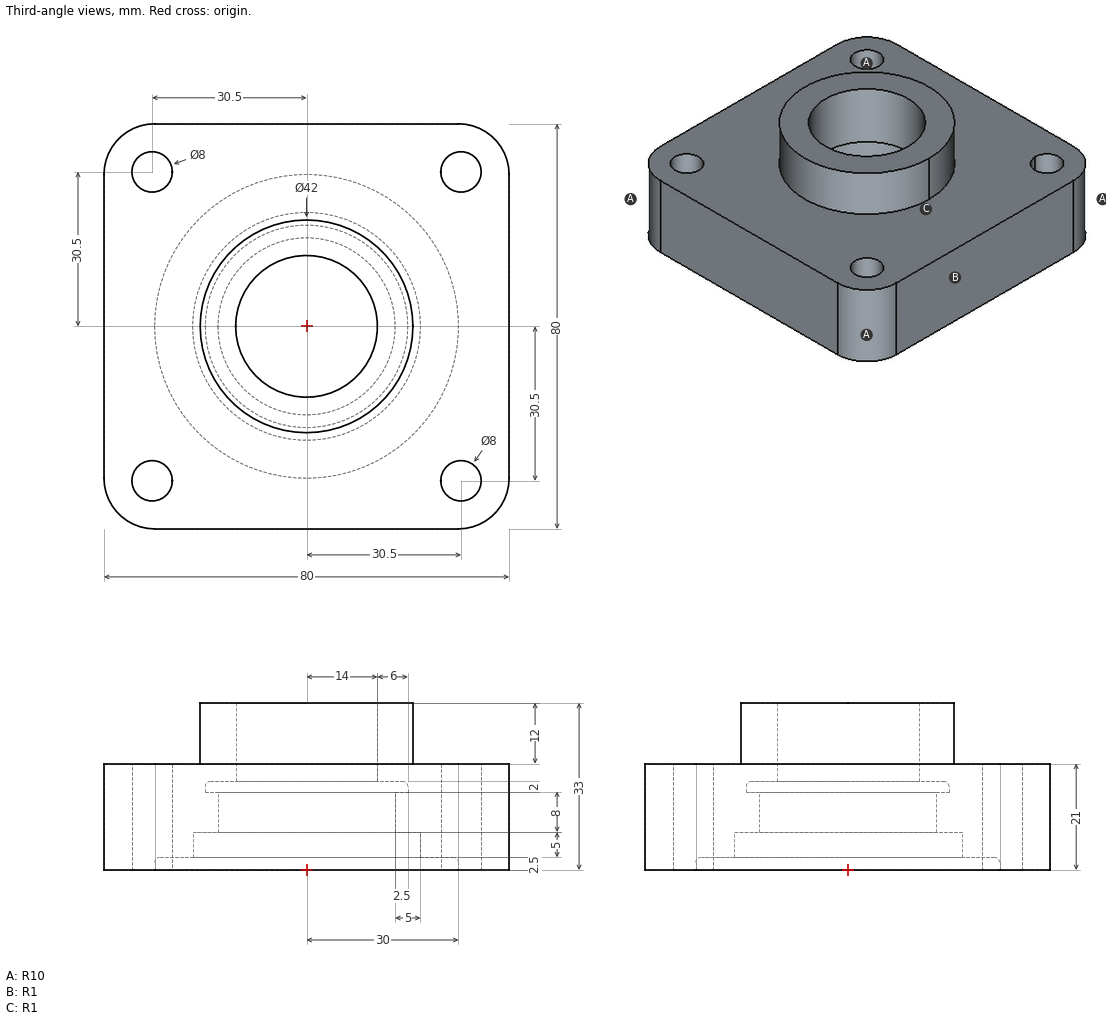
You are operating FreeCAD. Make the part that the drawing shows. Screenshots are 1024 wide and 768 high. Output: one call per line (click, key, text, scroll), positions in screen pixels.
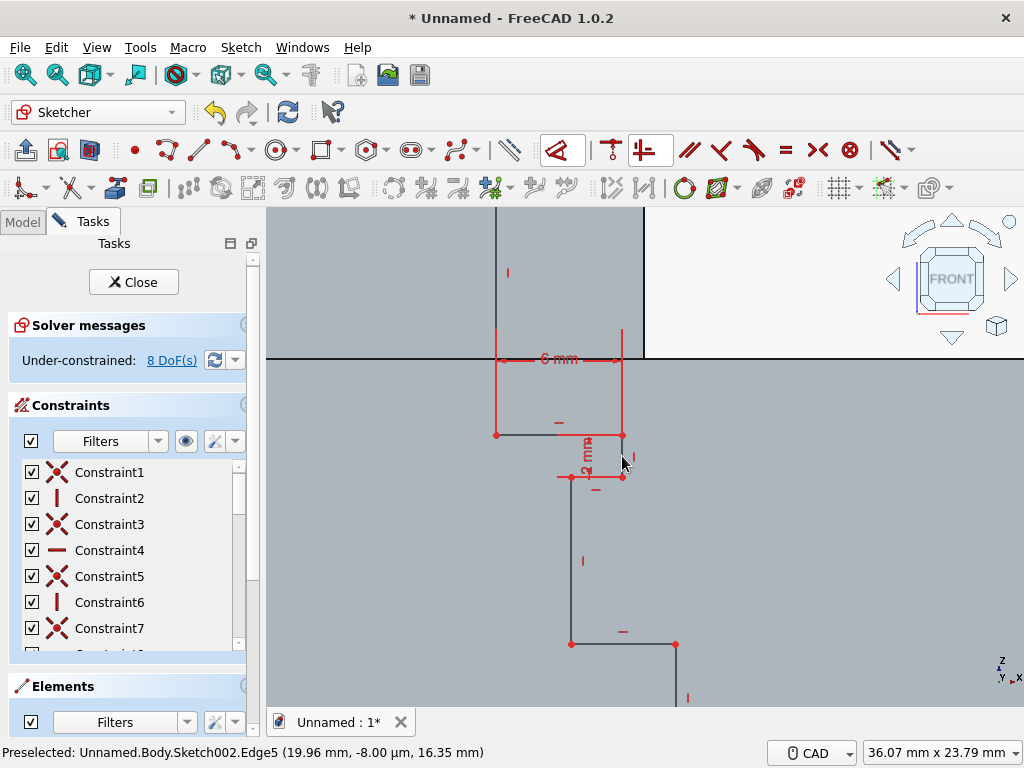
click(571, 527)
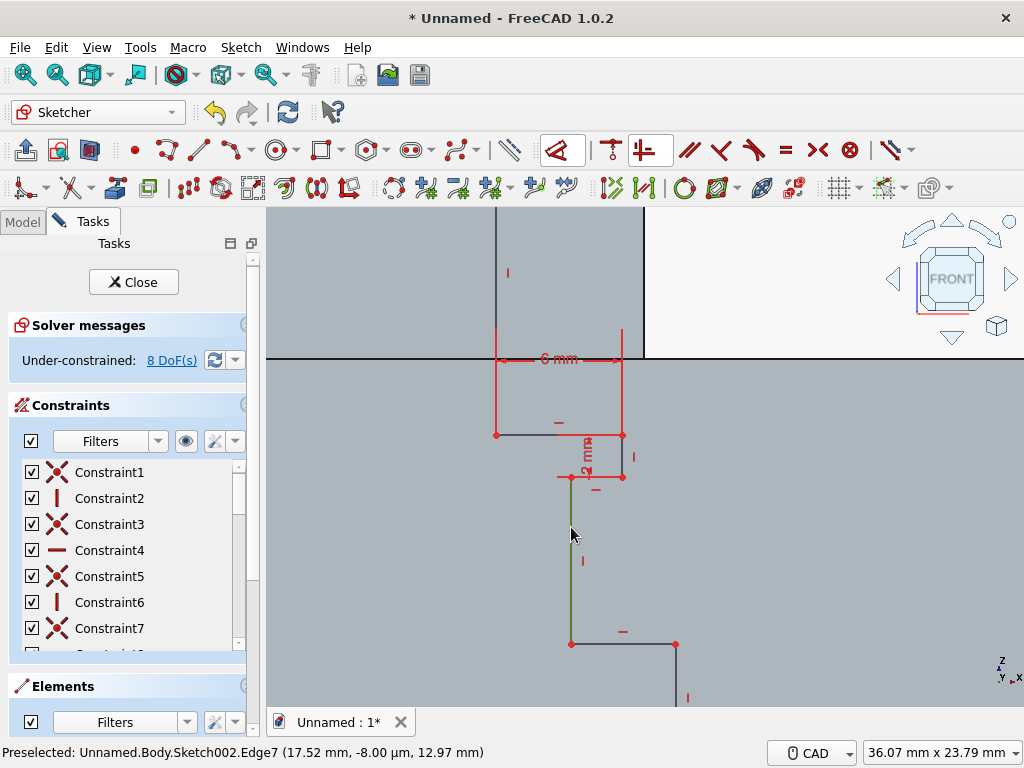
click(580, 150)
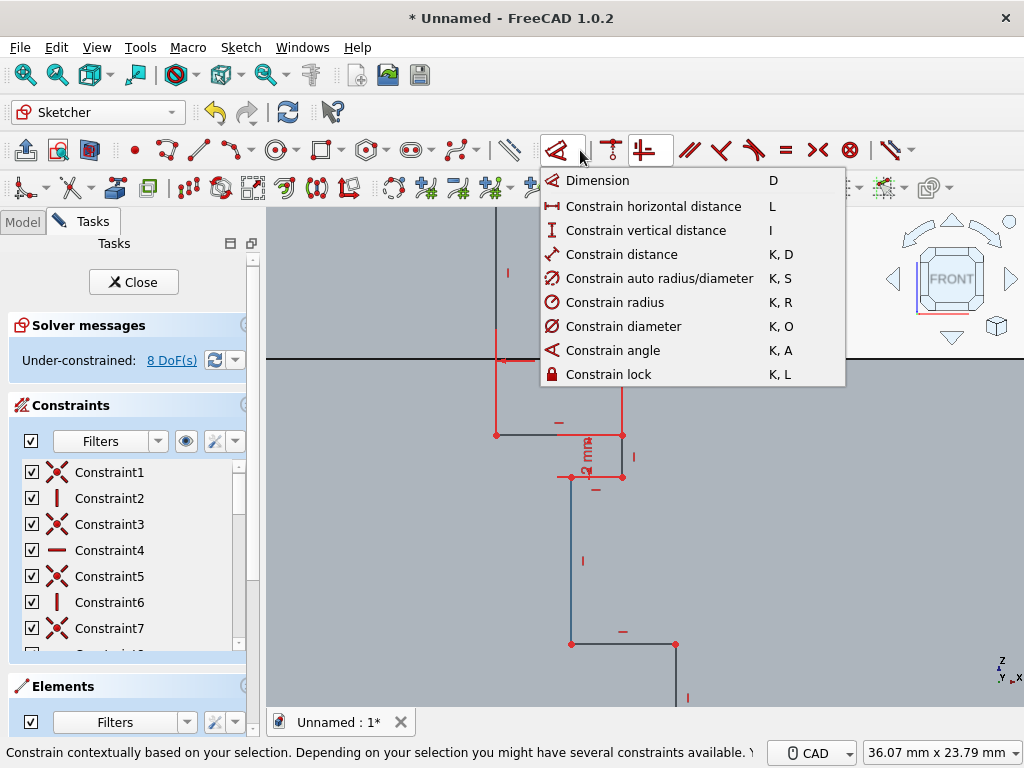
click(693, 230)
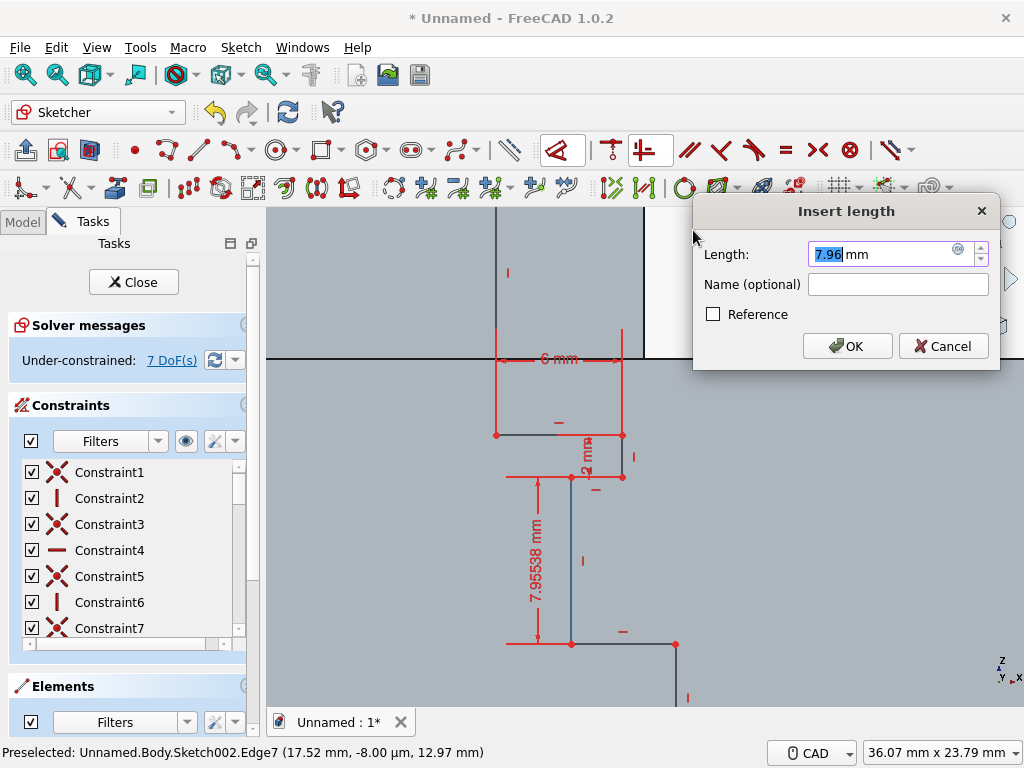
text(8)
key(Return)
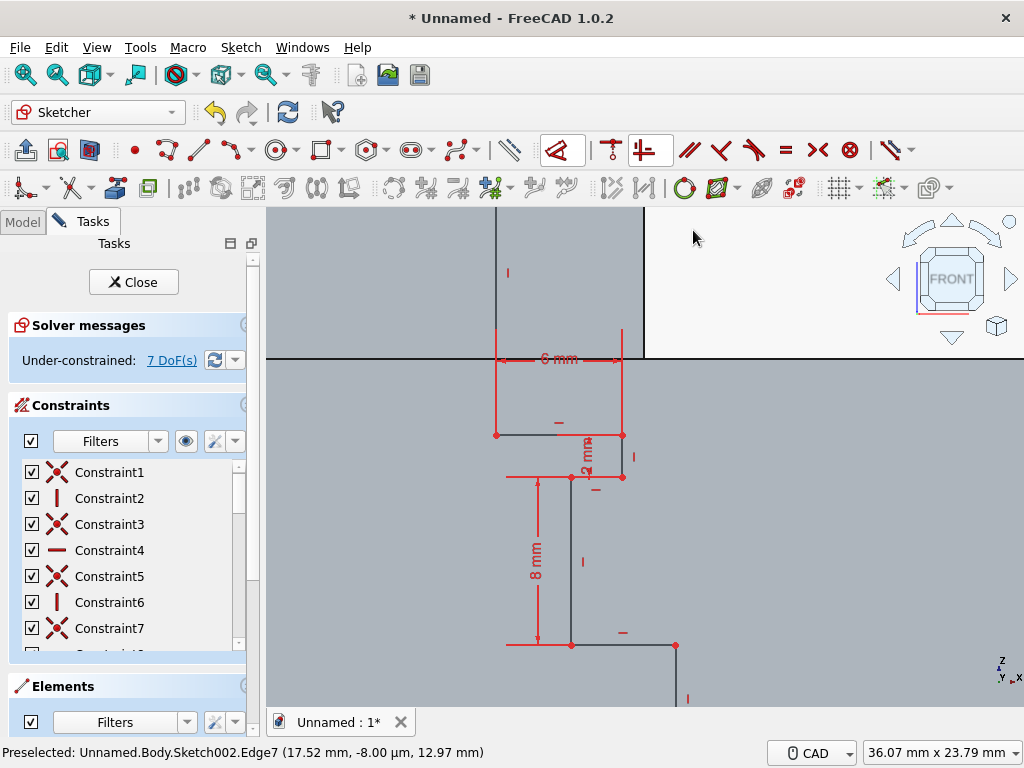
click(603, 645)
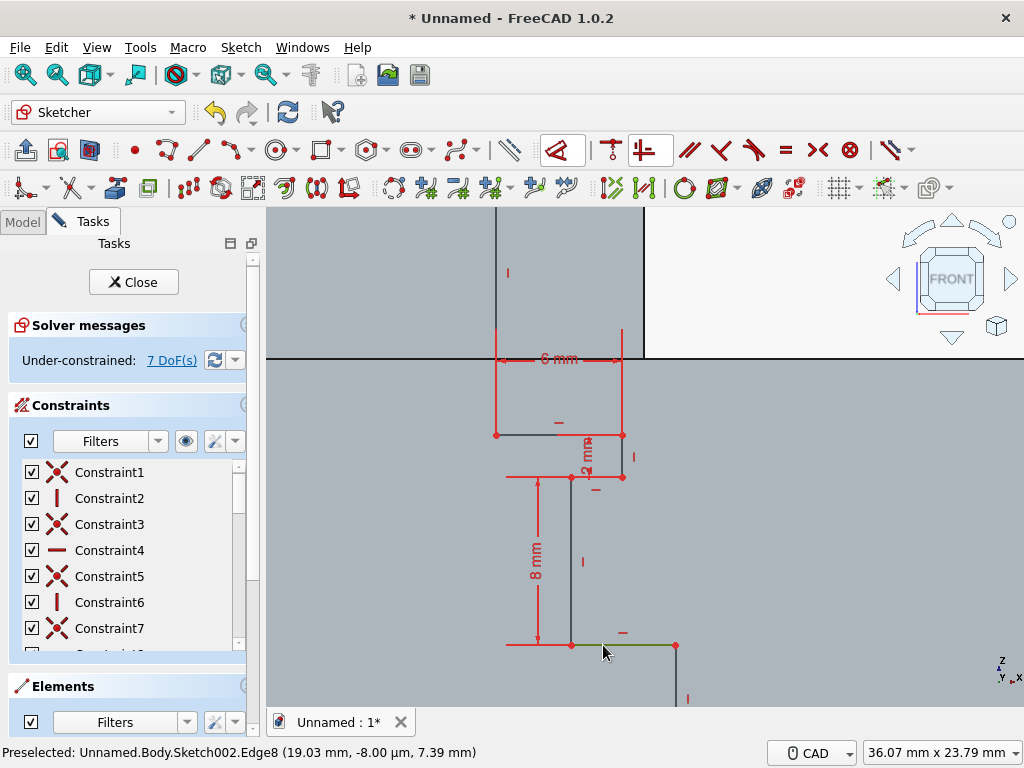
key(l)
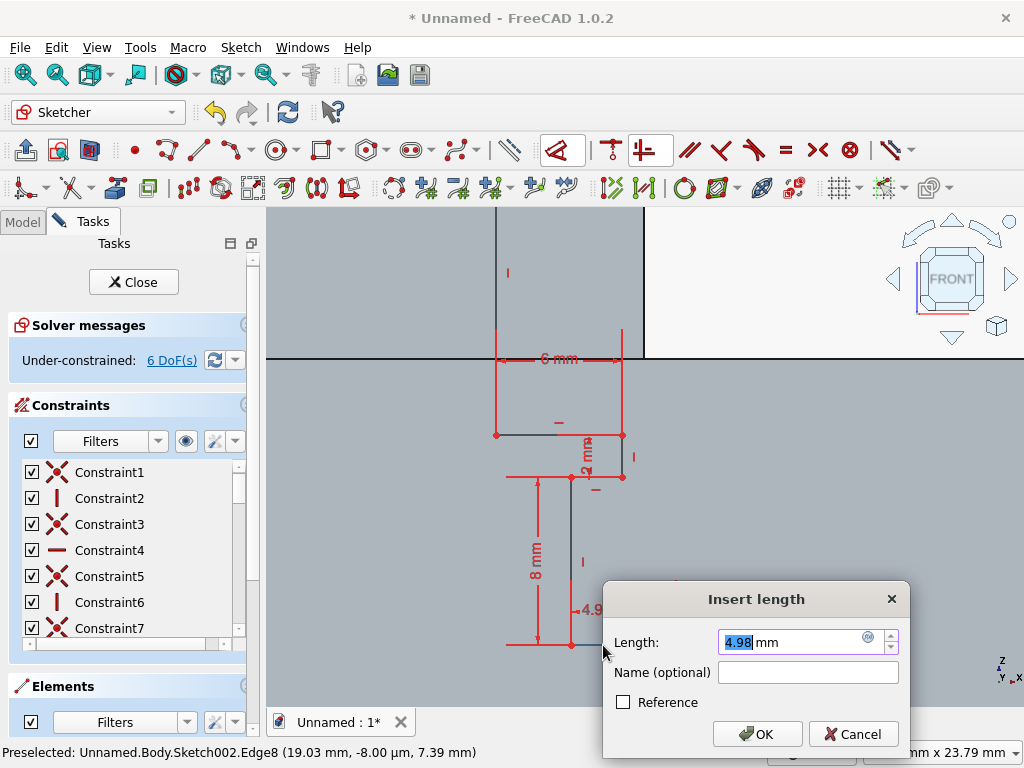
text(5)
key(Return)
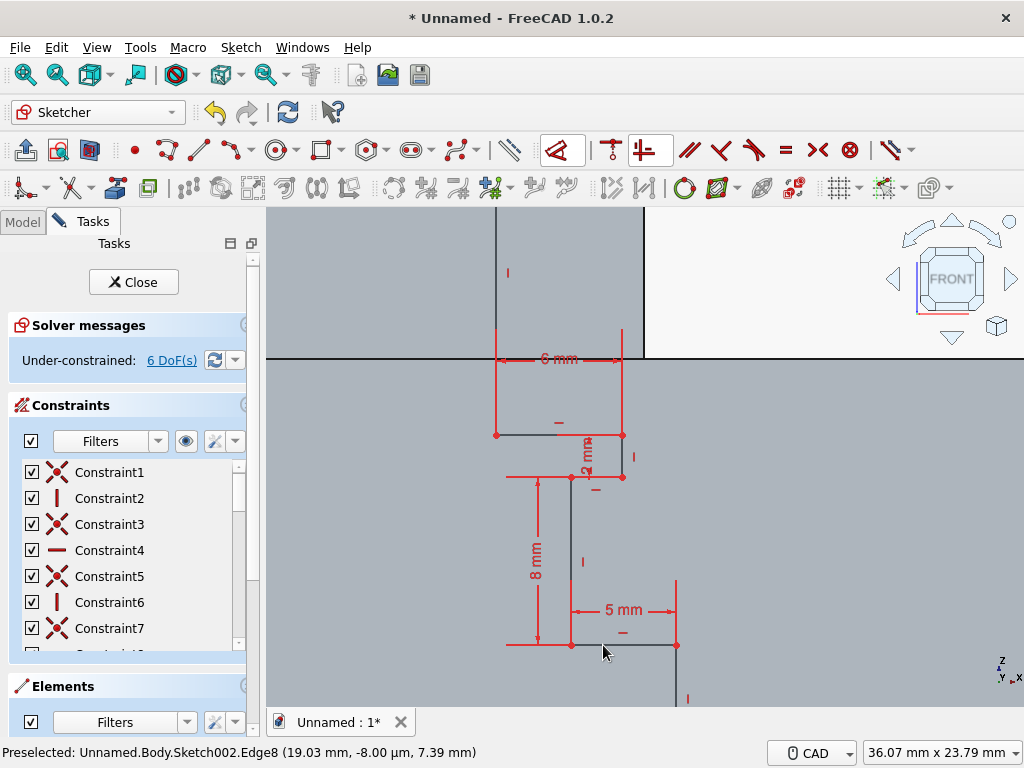
click(676, 677)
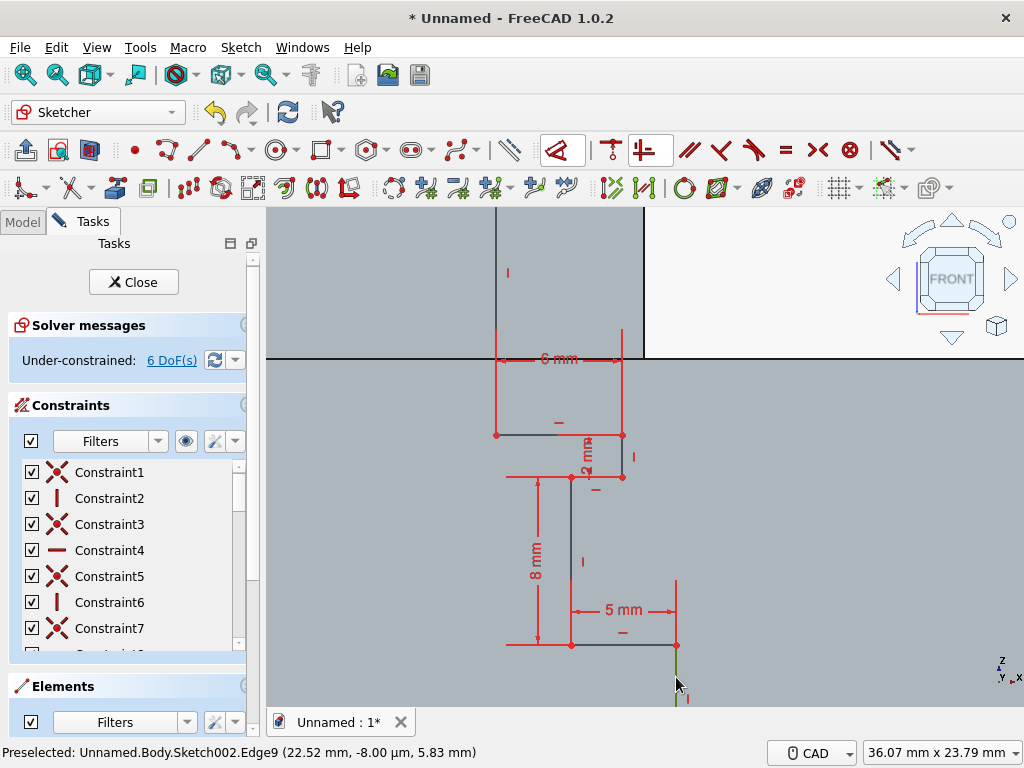
key(i)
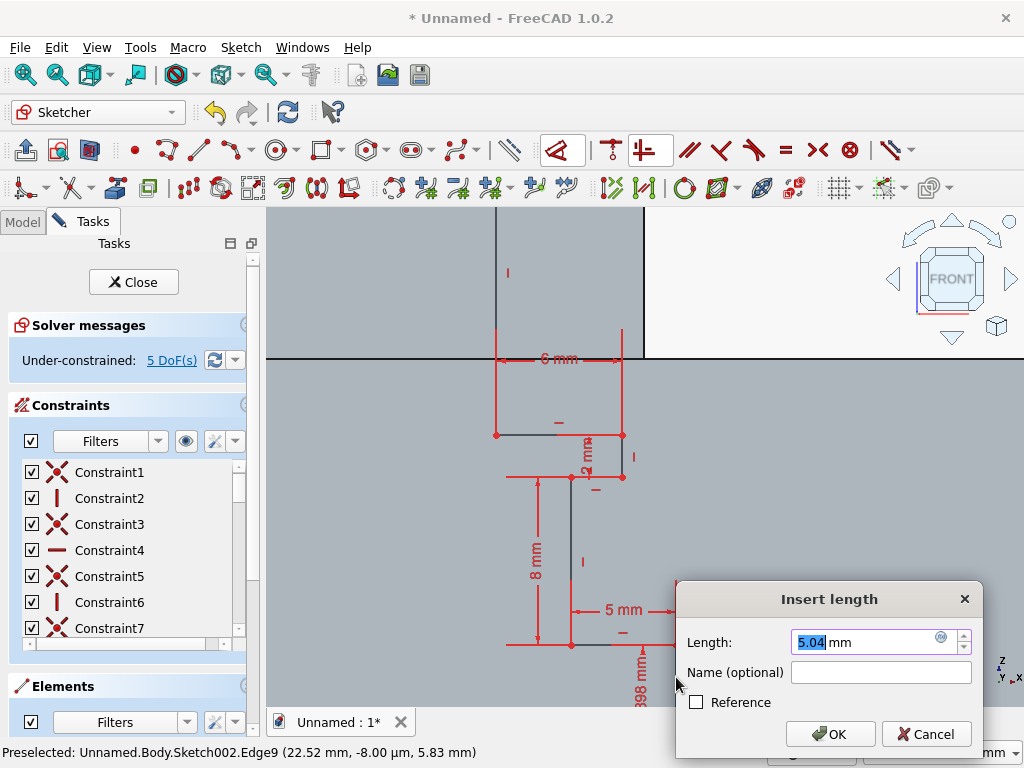
text(5)
key(Return)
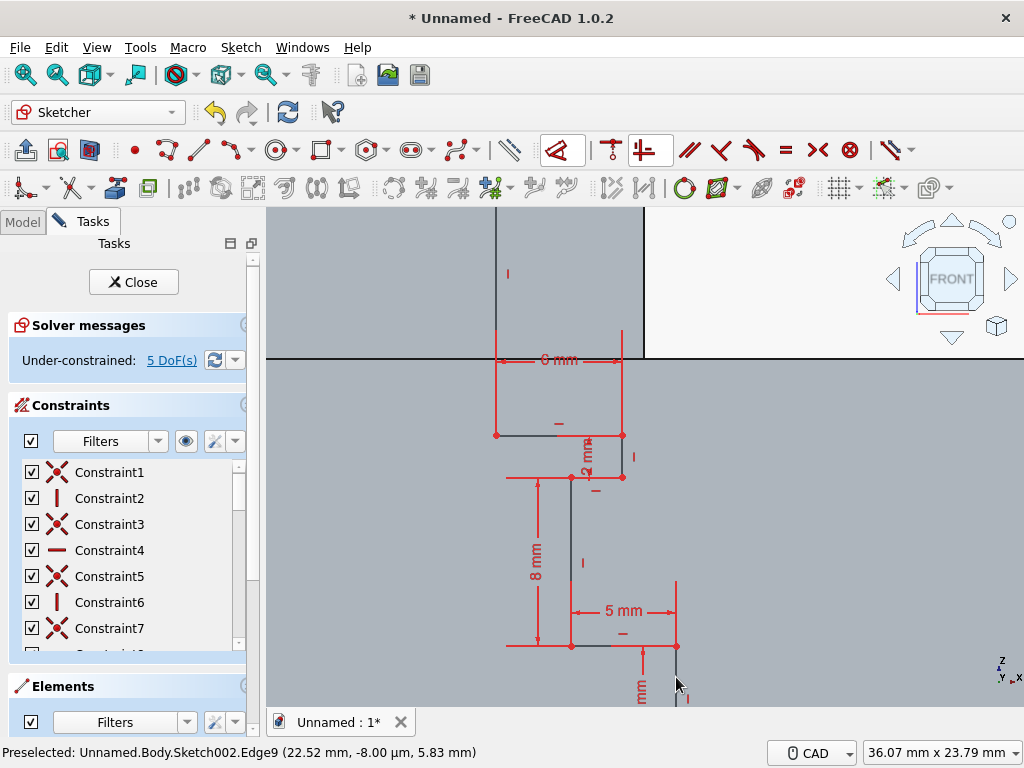
scroll(624, 460, down, 4)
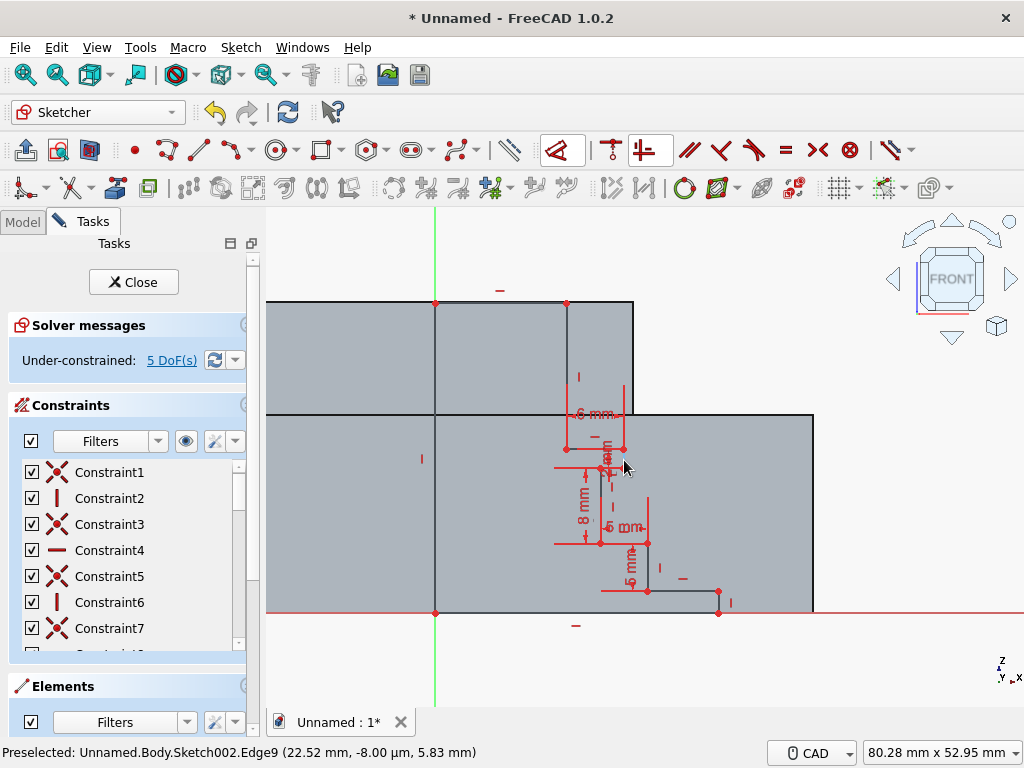
click(435, 520)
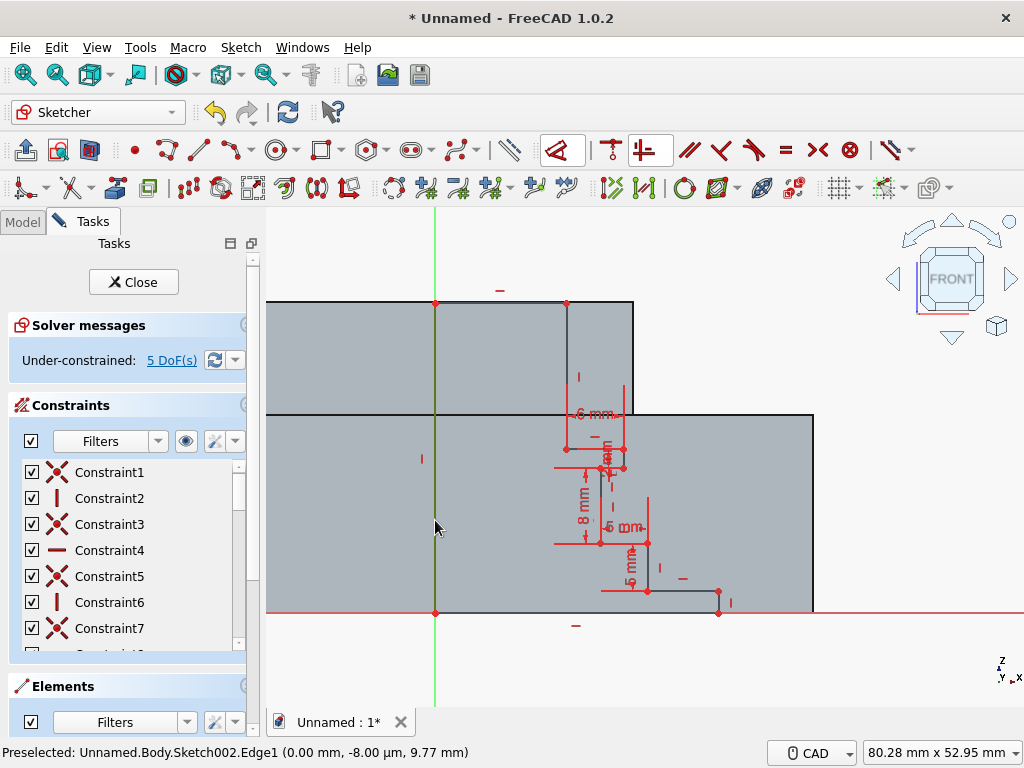
click(580, 150)